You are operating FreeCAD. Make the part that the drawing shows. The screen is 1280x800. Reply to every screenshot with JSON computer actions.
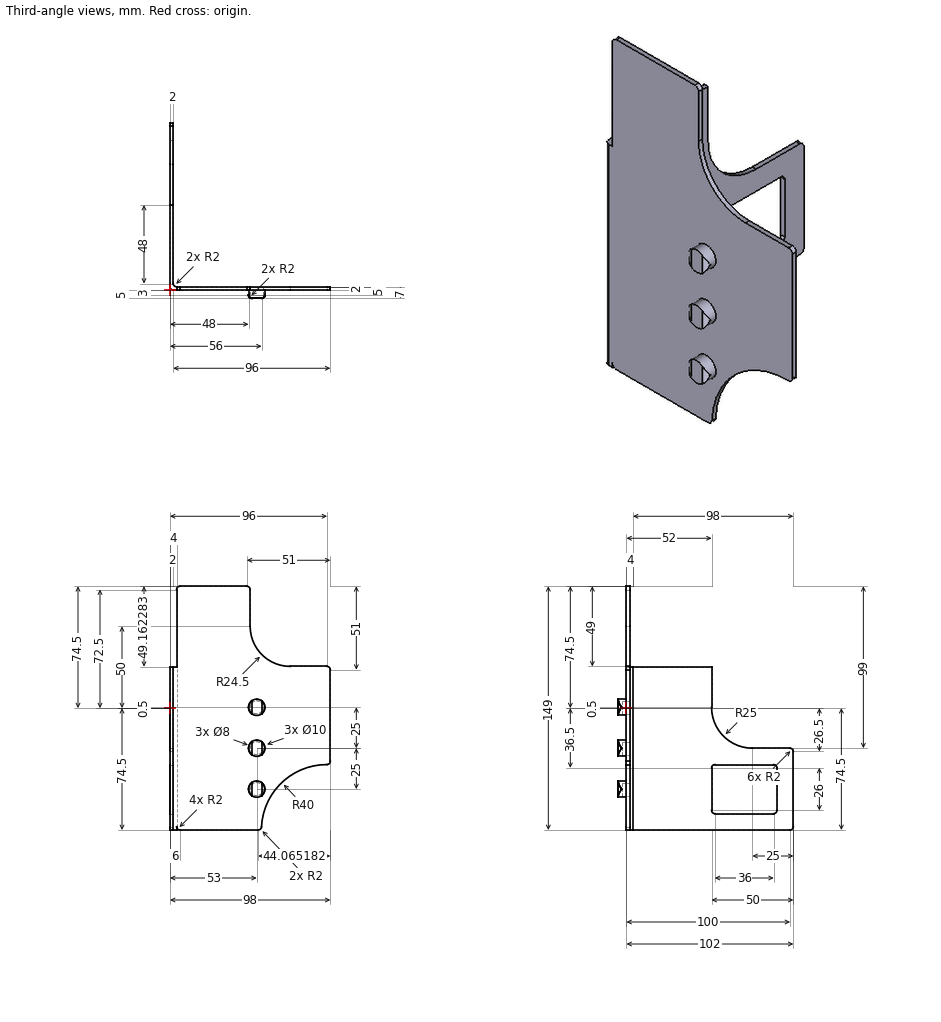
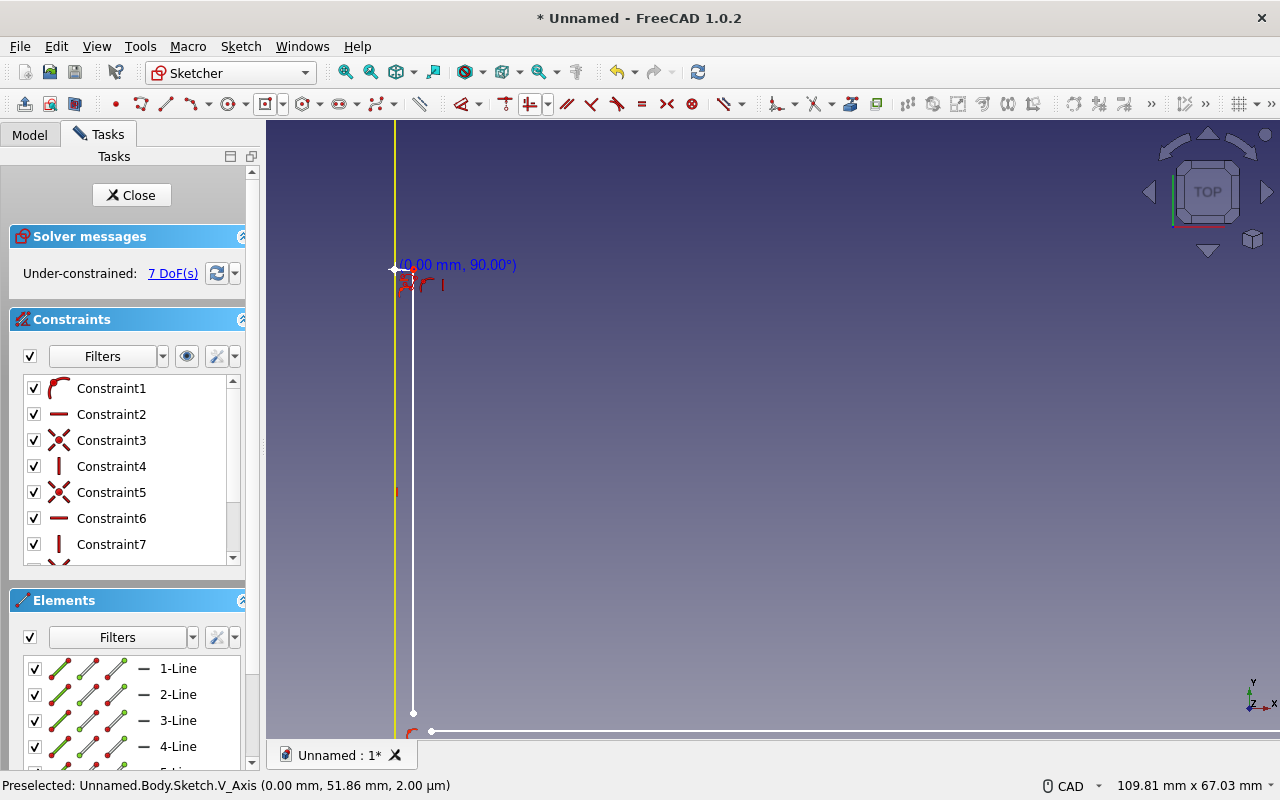
{"action": "scroll", "coordinate": [414, 268], "scroll_direction": "down", "scroll_amount": 2}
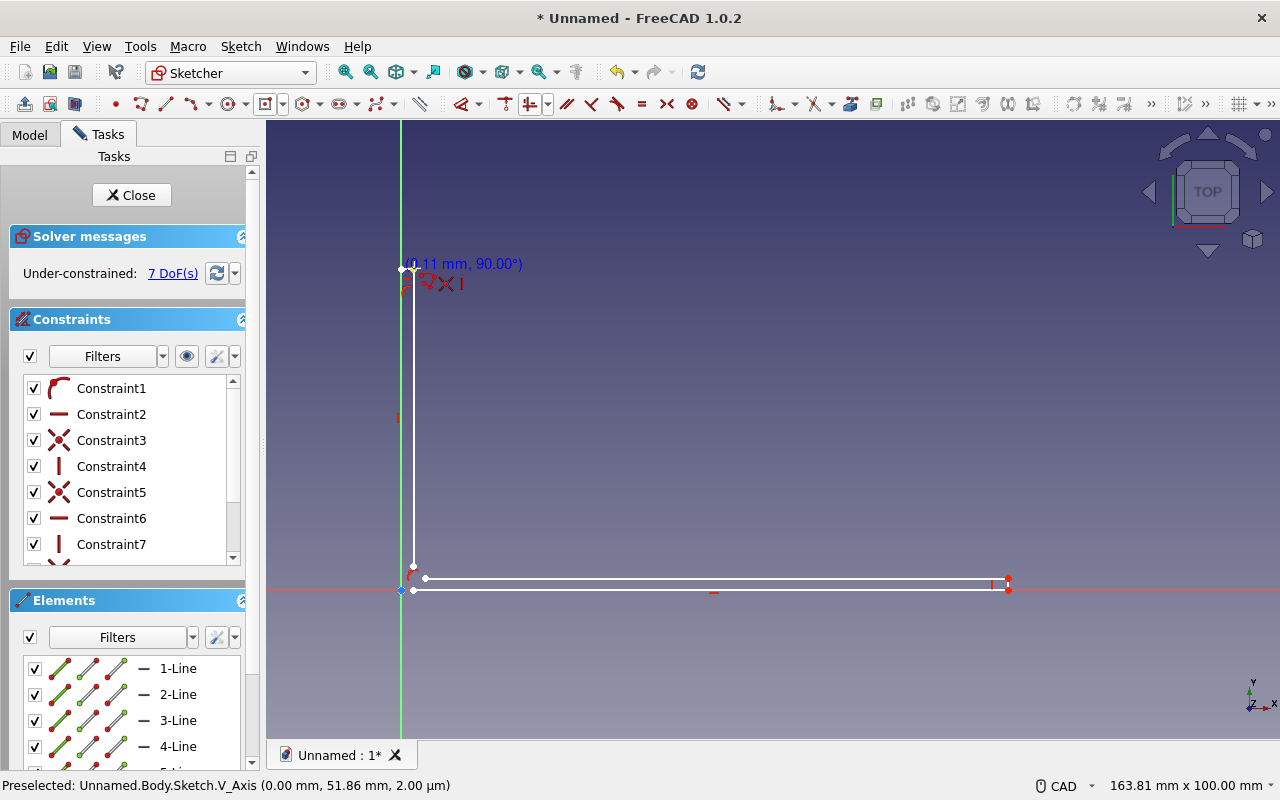
{"action": "scroll", "coordinate": [401, 578], "scroll_direction": "up", "scroll_amount": 2}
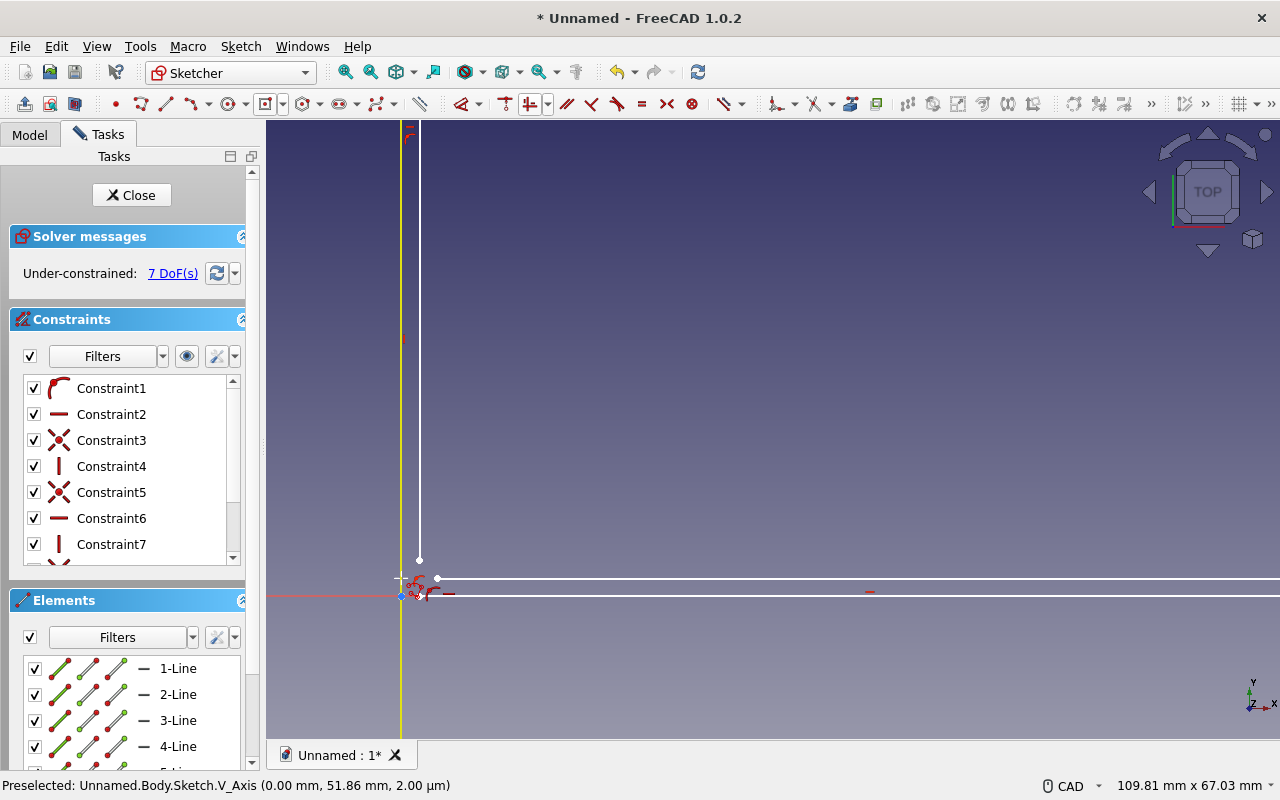
{"action": "left_click", "coordinate": [410, 578]}
{"action": "right_click", "coordinate": [410, 578]}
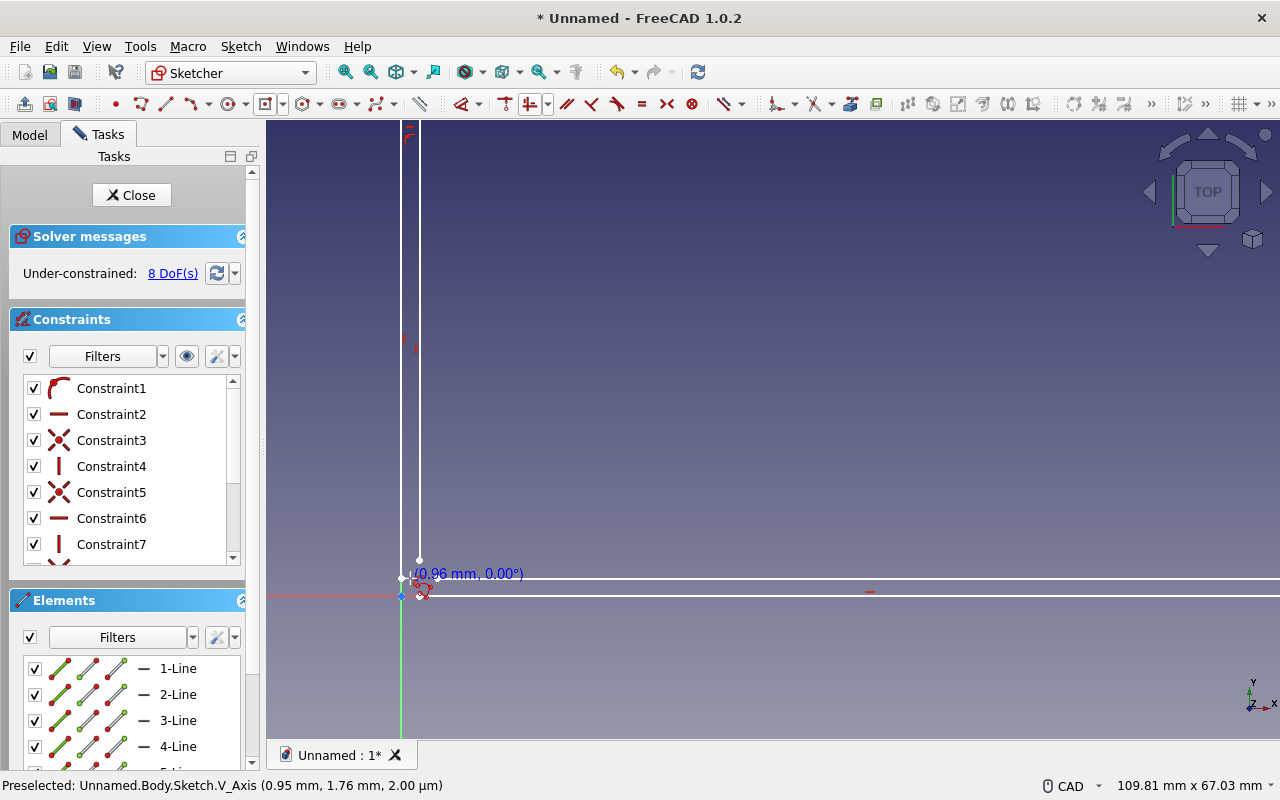
{"action": "key", "text": "g 3 a"}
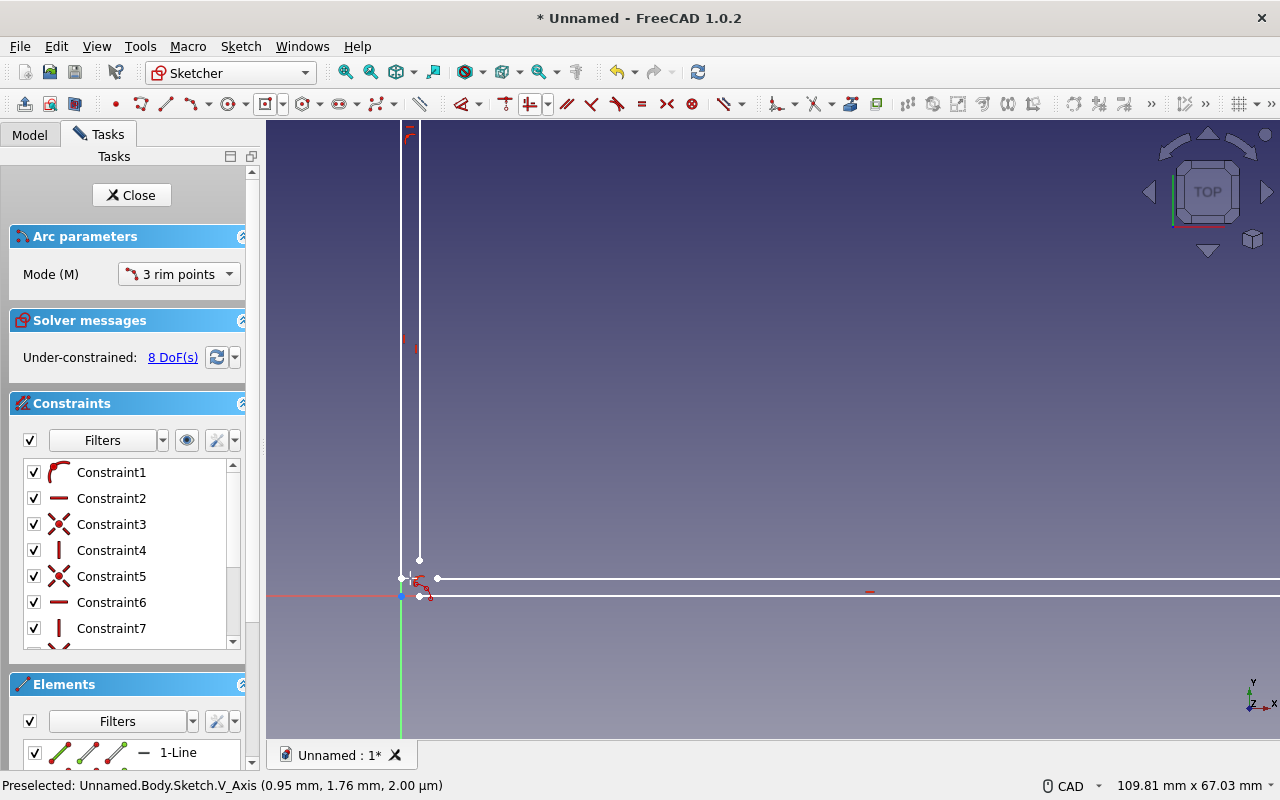
{"action": "left_click", "coordinate": [438, 579]}
{"action": "left_click", "coordinate": [420, 561]}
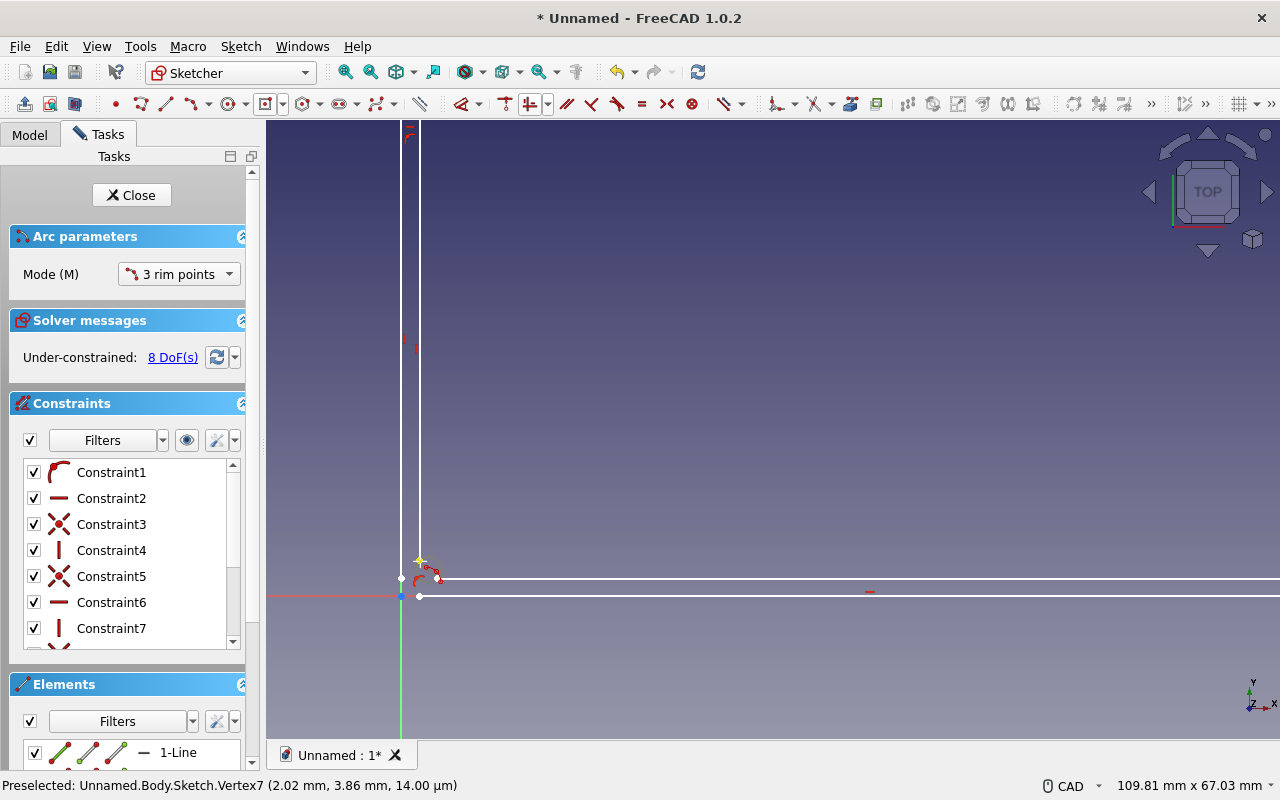
{"action": "scroll", "coordinate": [425, 572], "scroll_direction": "up", "scroll_amount": 6}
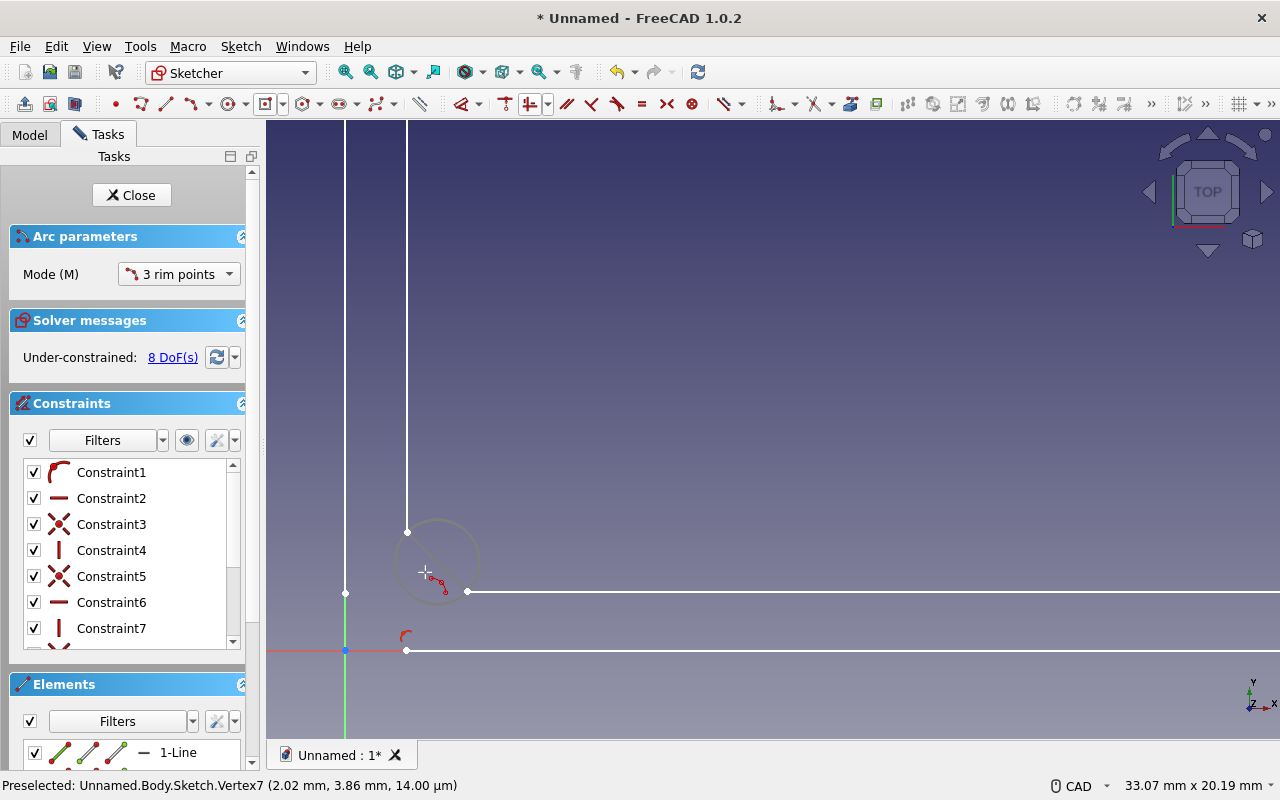
{"action": "left_click", "coordinate": [425, 571]}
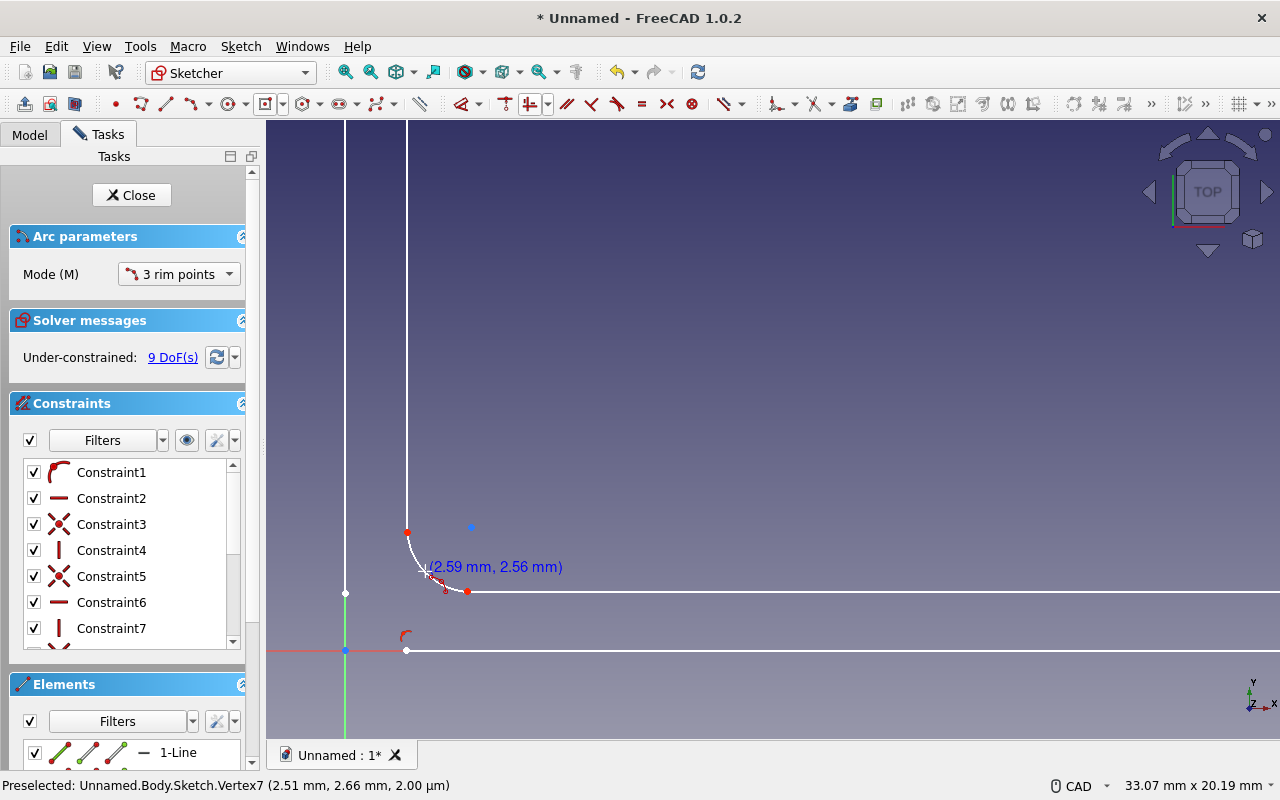
{"action": "scroll", "coordinate": [415, 575], "scroll_direction": "down", "scroll_amount": 8}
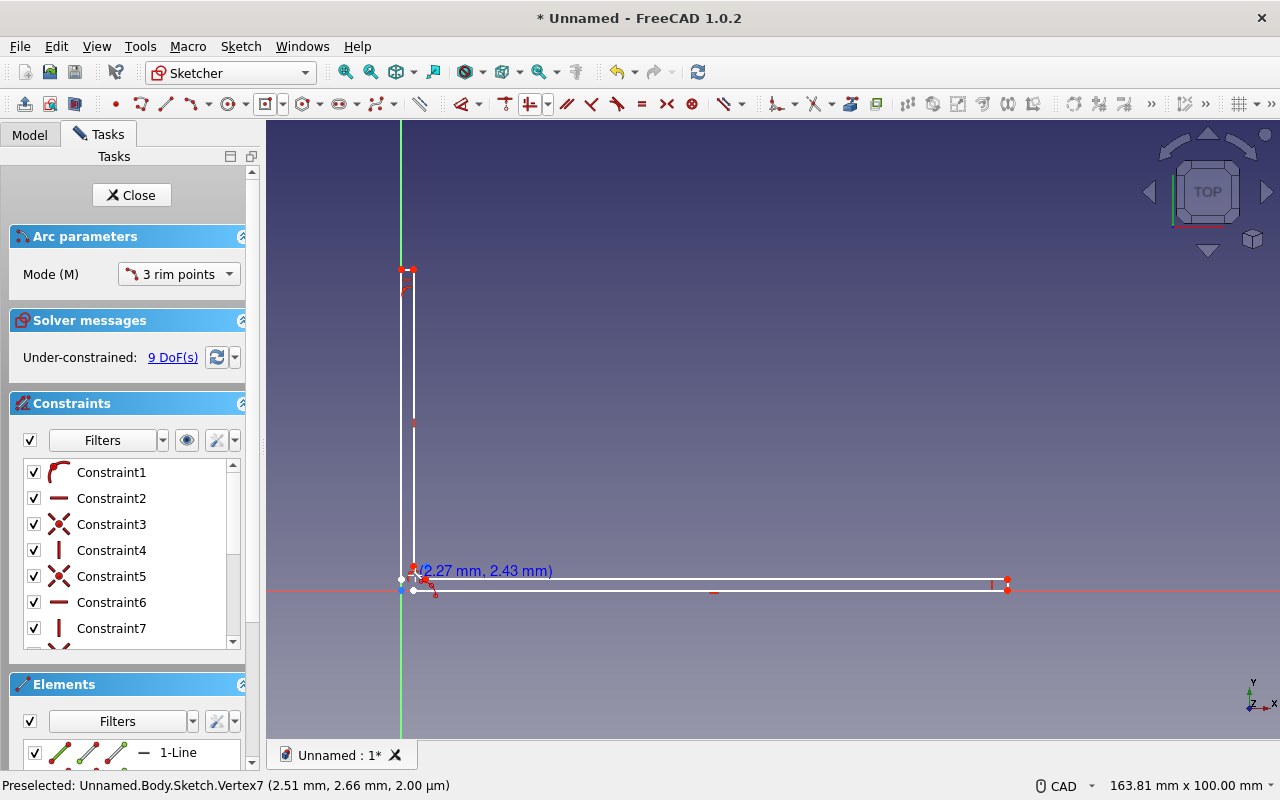
{"action": "scroll", "coordinate": [401, 578], "scroll_direction": "up", "scroll_amount": 2}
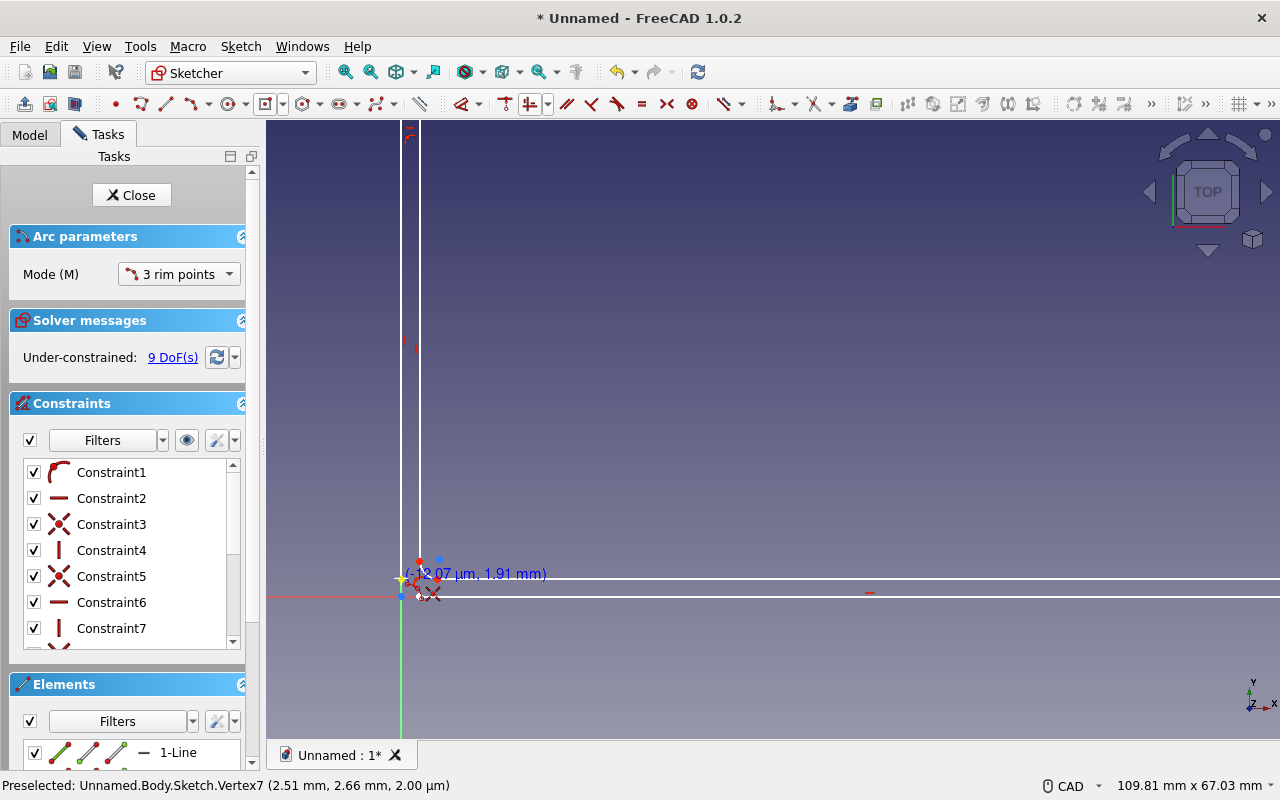
{"action": "left_click", "coordinate": [401, 580]}
{"action": "left_click", "coordinate": [419, 597]}